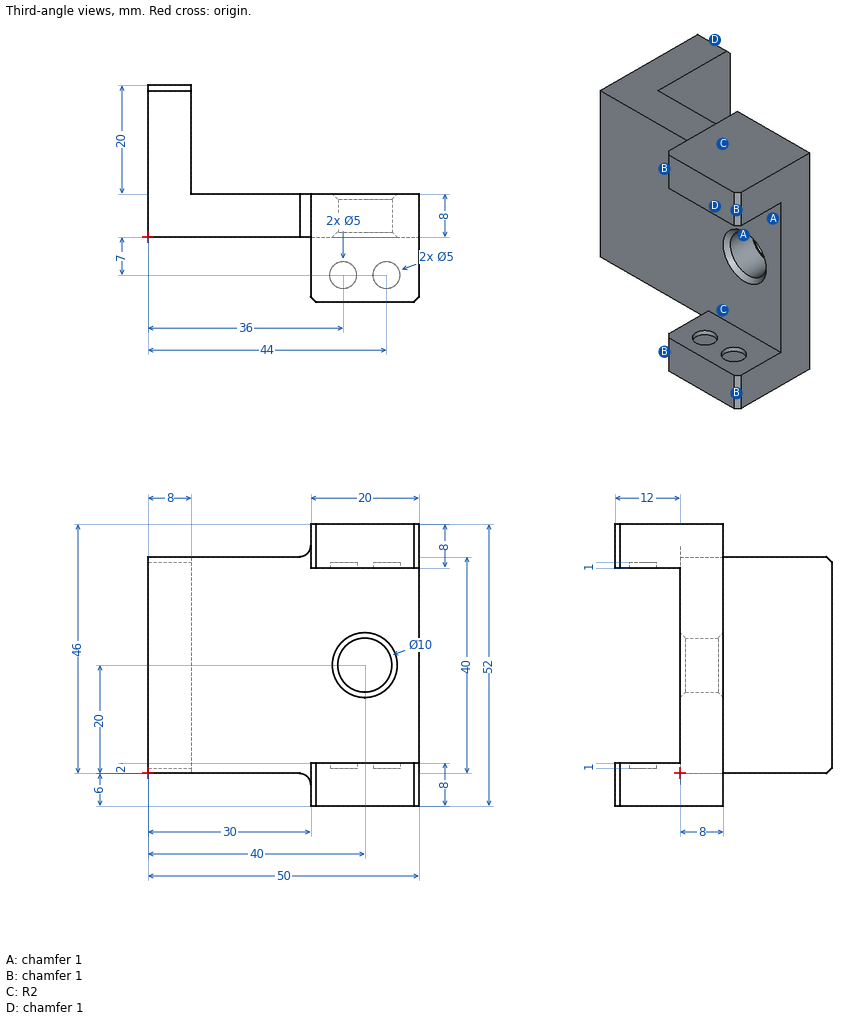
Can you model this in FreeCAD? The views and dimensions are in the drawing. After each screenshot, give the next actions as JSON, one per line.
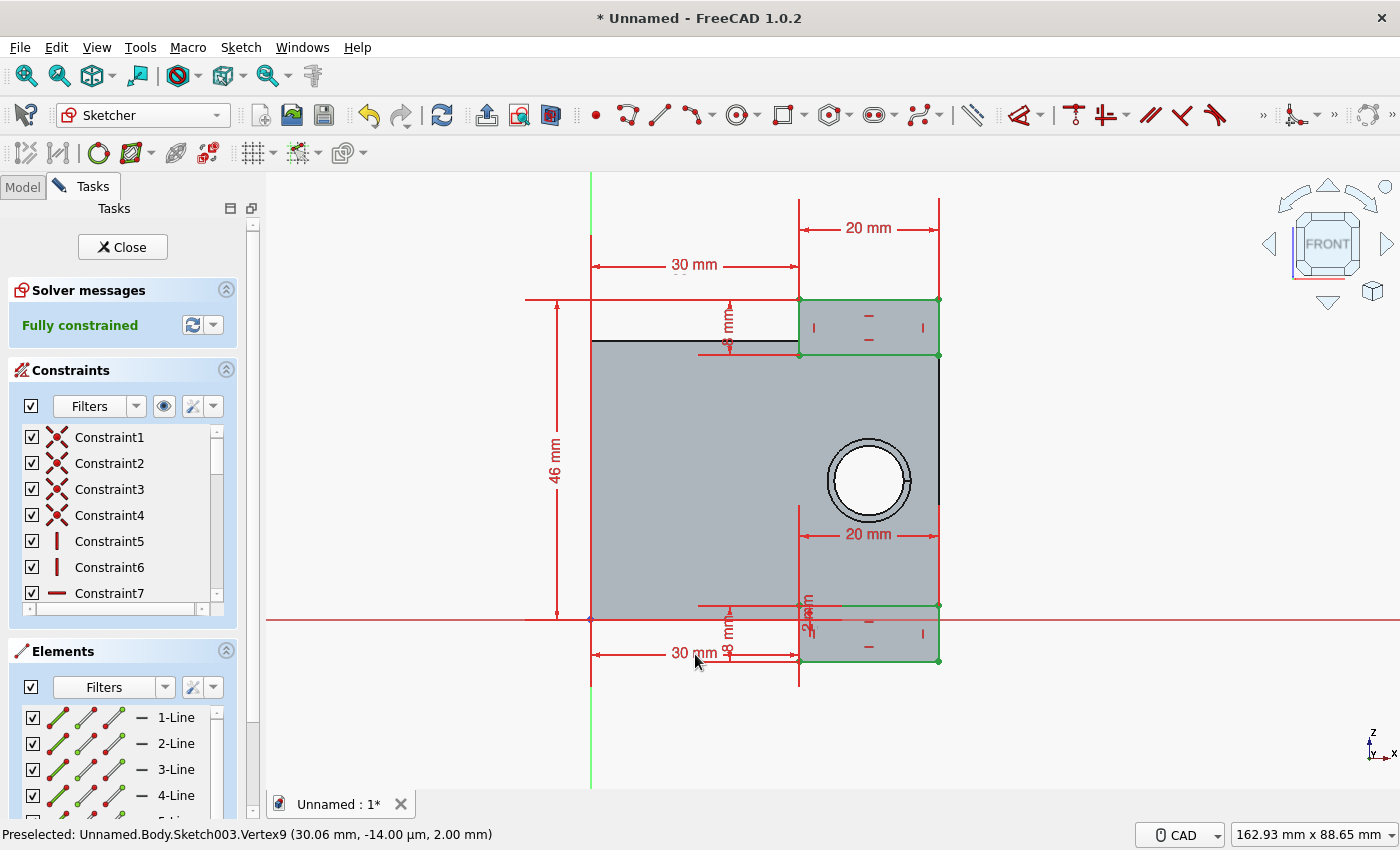
{"action": "left_click", "coordinate": [123, 247]}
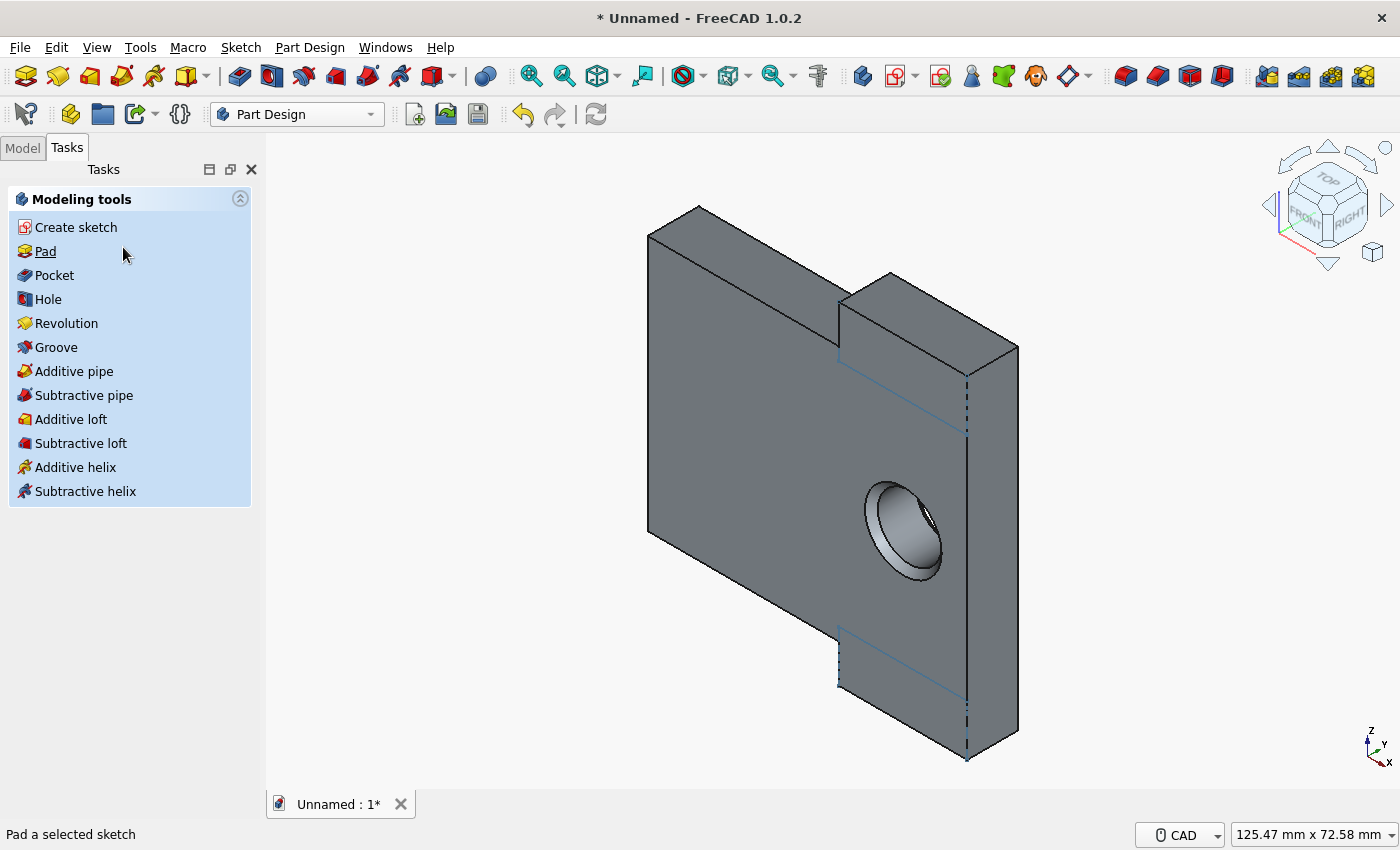
{"action": "left_click", "coordinate": [26, 76]}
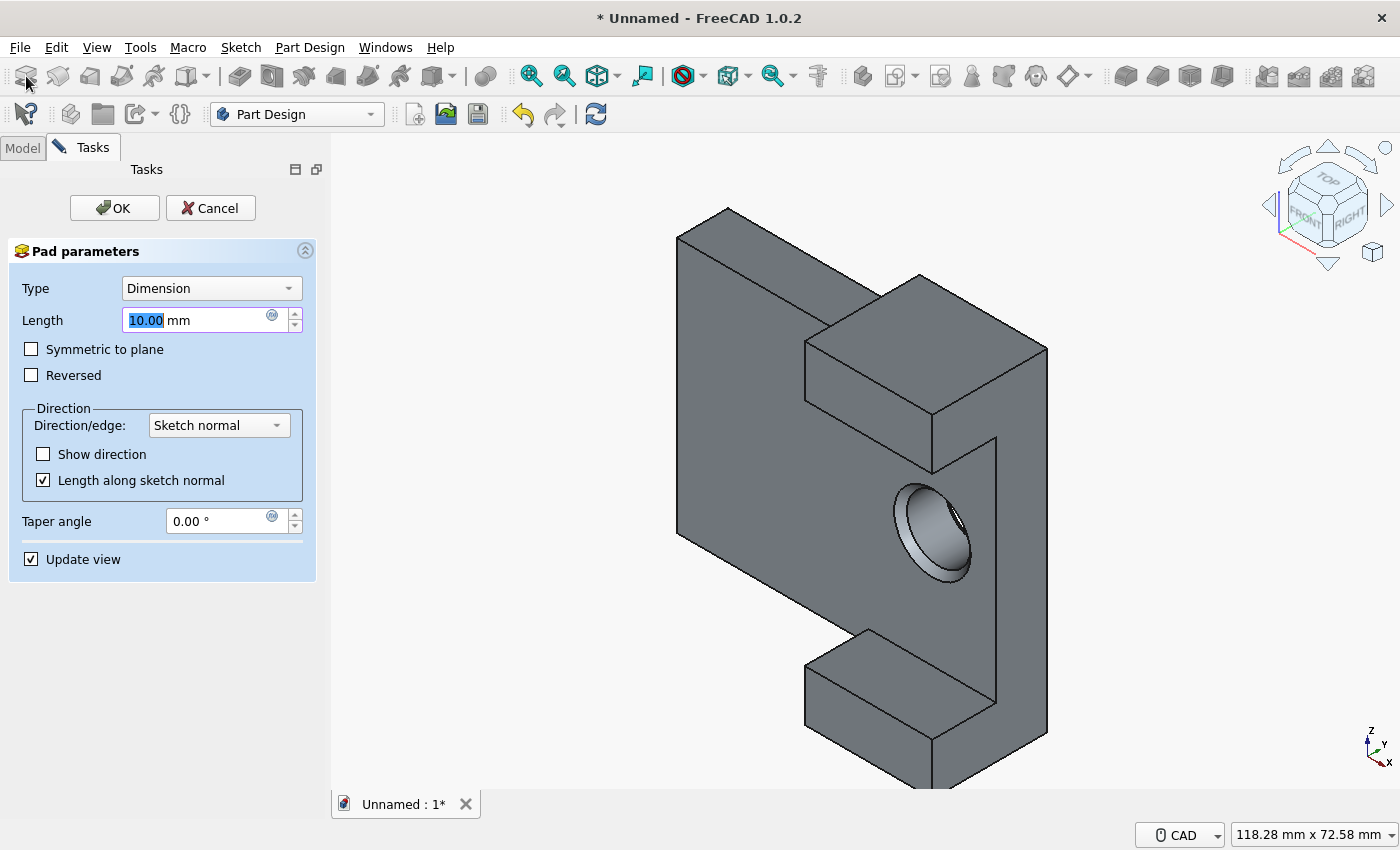
{"action": "type", "text": "12"}
{"action": "key", "text": "Tab"}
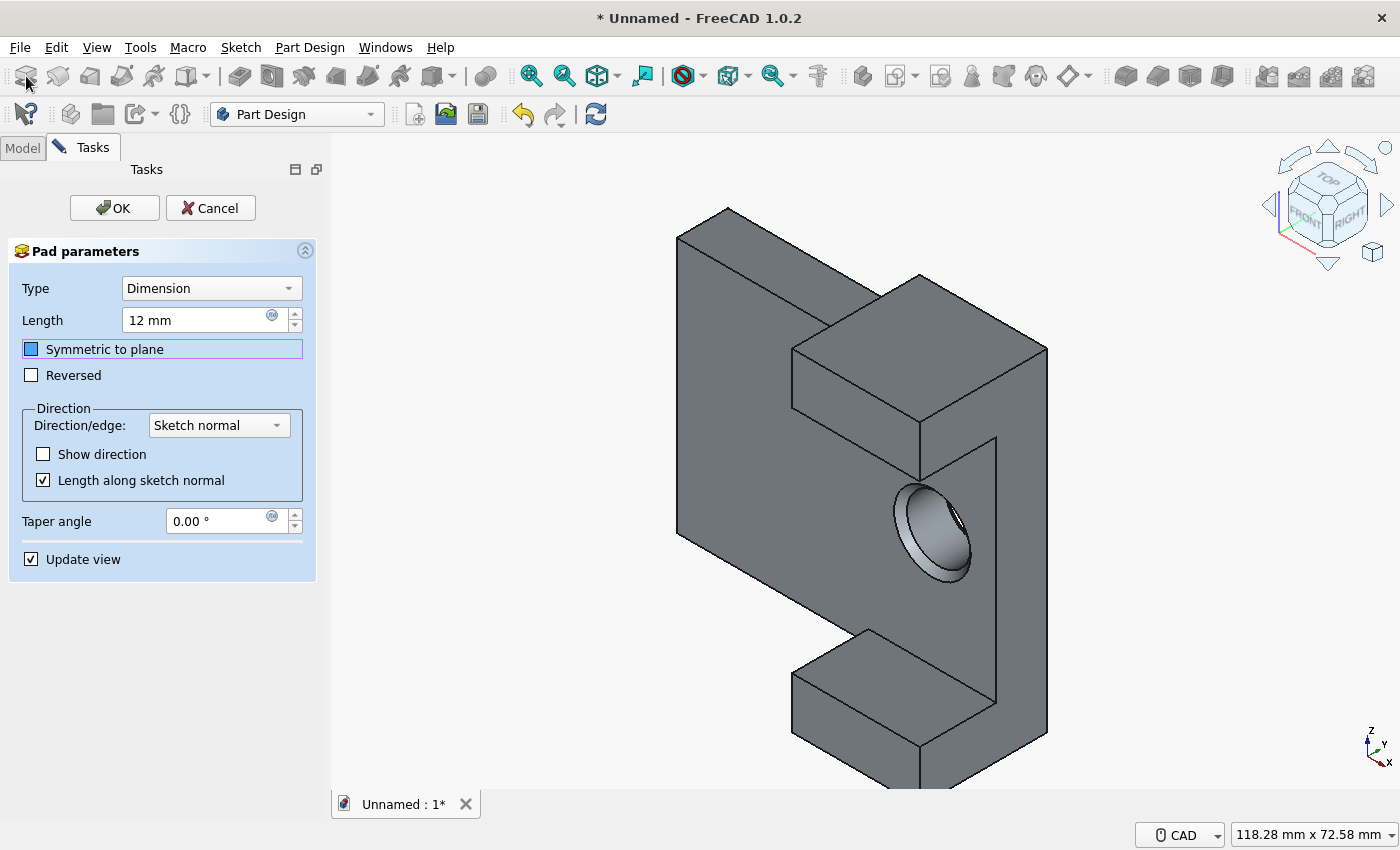
{"action": "left_click", "coordinate": [115, 208]}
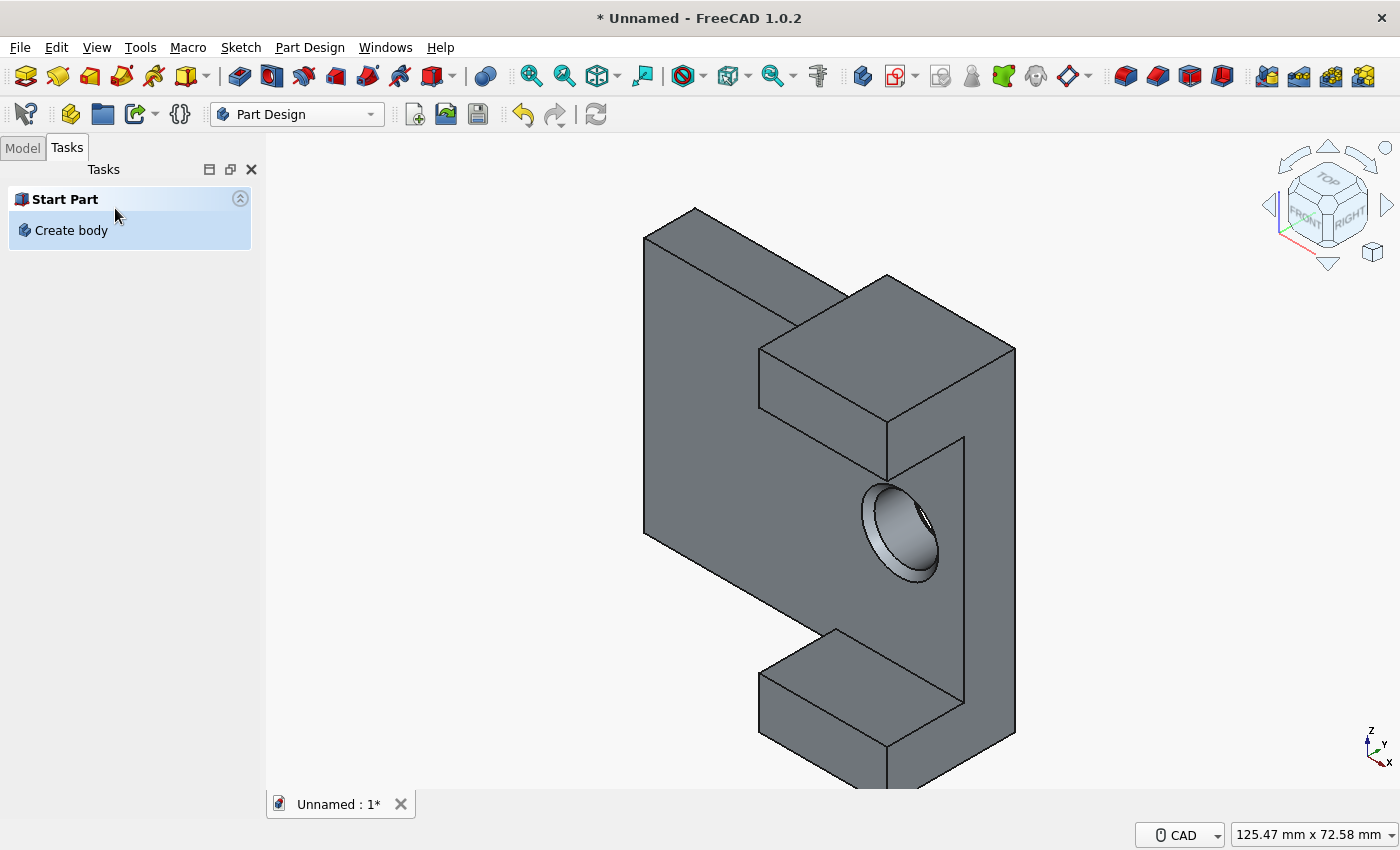
{"action": "left_click", "coordinate": [532, 76]}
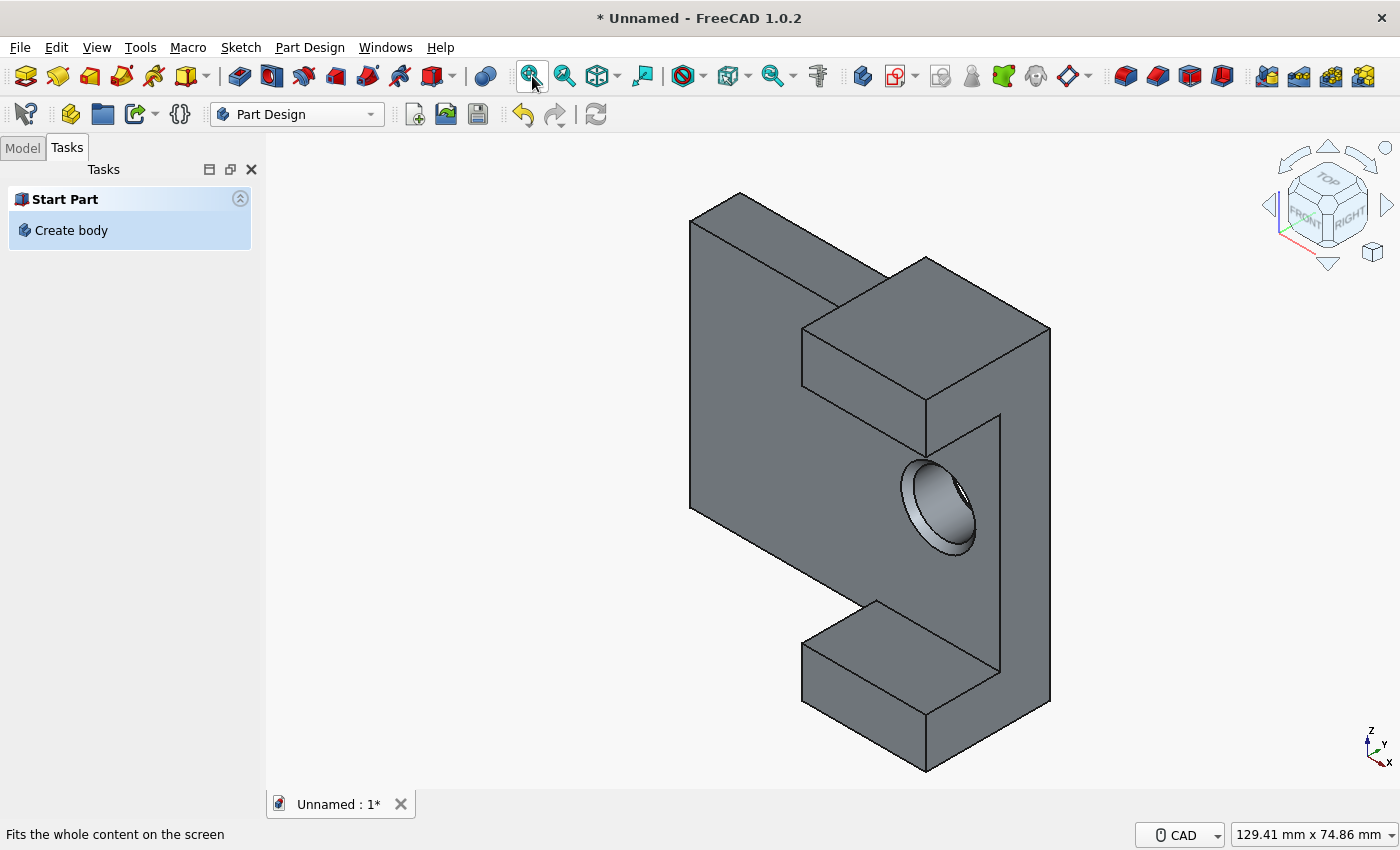
{"action": "left_click", "coordinate": [926, 428]}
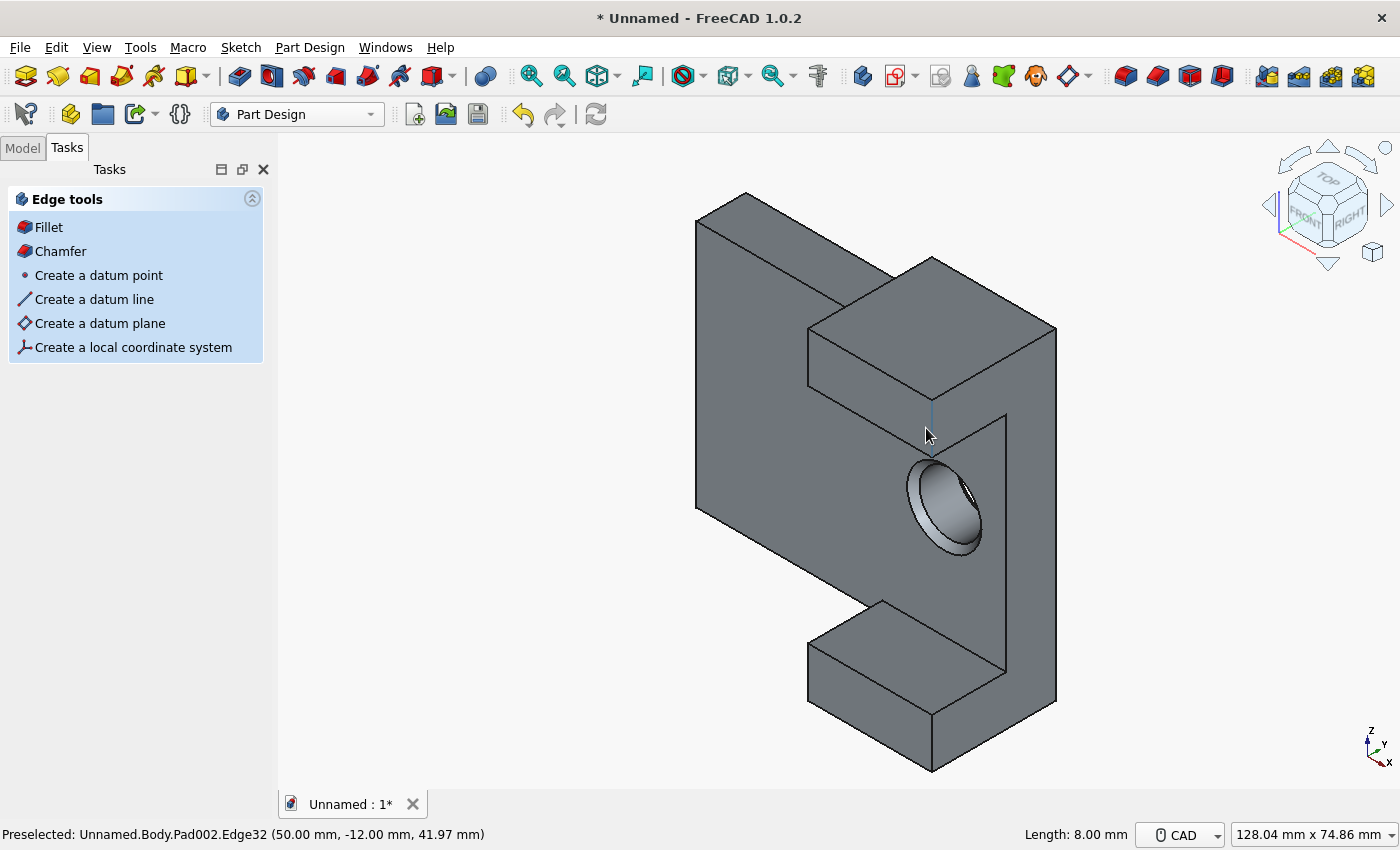
{"action": "left_click", "coordinate": [932, 743], "text": "ctrl"}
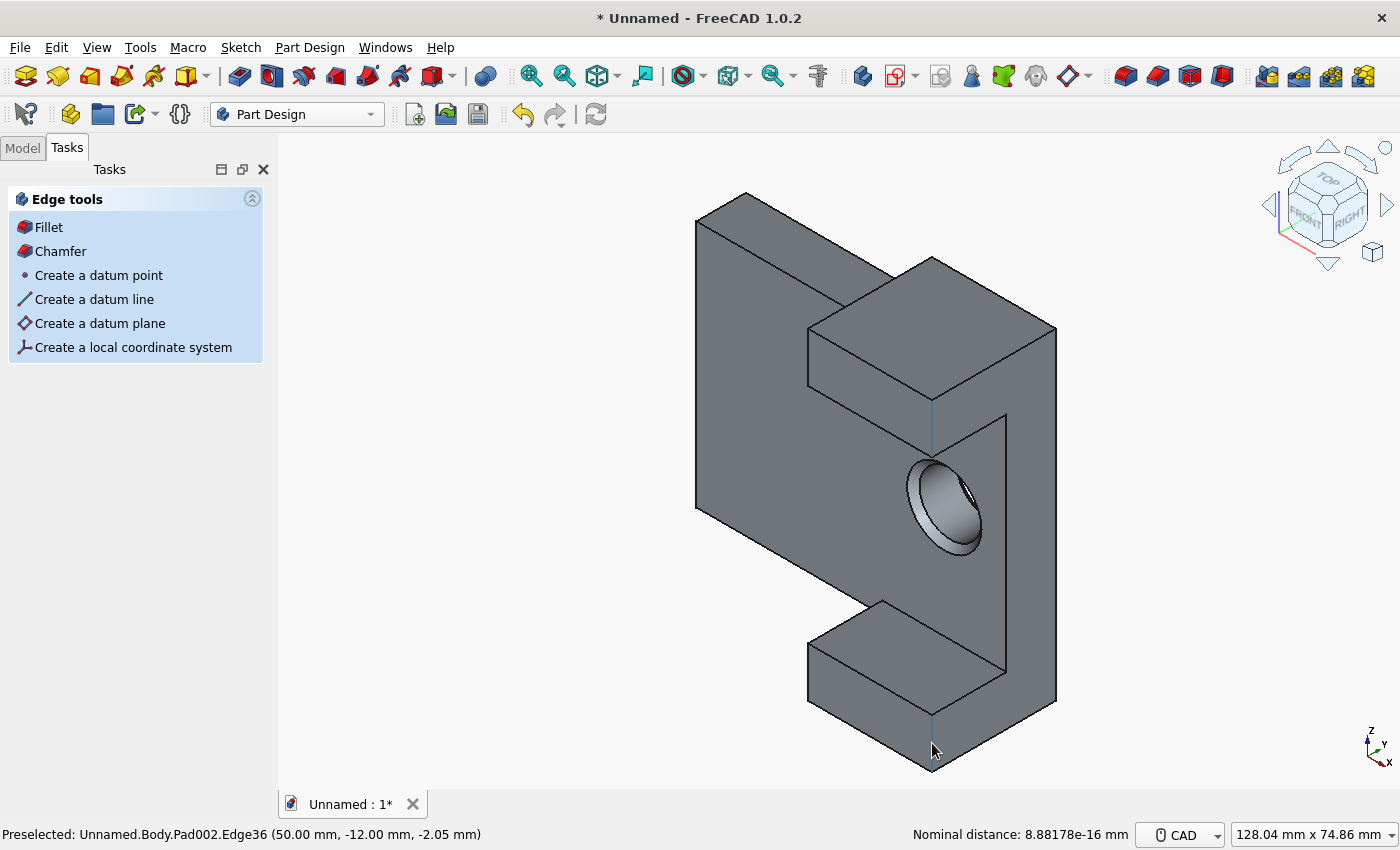
{"action": "key", "text": "2"}